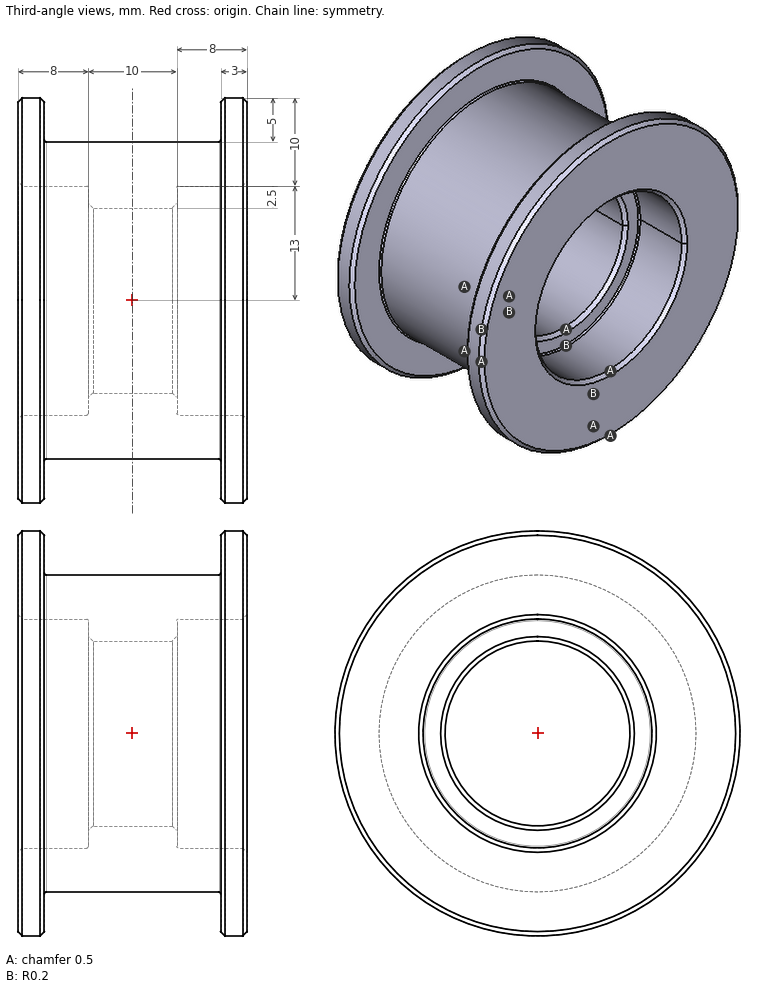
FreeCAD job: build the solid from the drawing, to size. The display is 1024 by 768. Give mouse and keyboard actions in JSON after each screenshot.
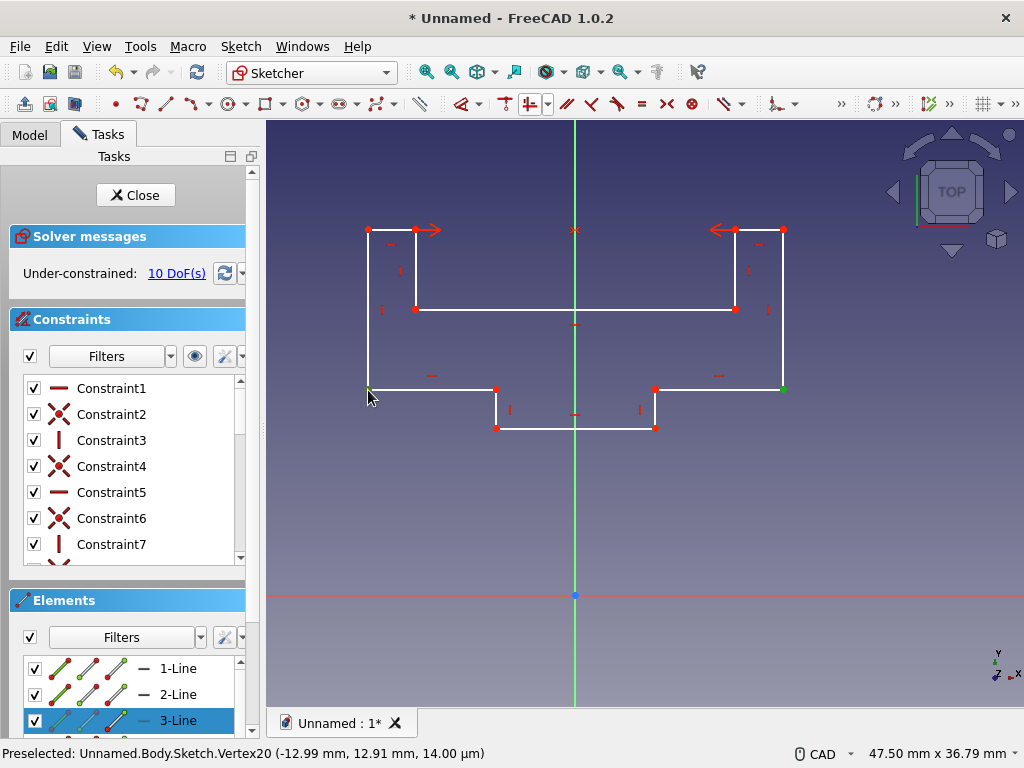
{"action": "left_click", "coordinate": [575, 641]}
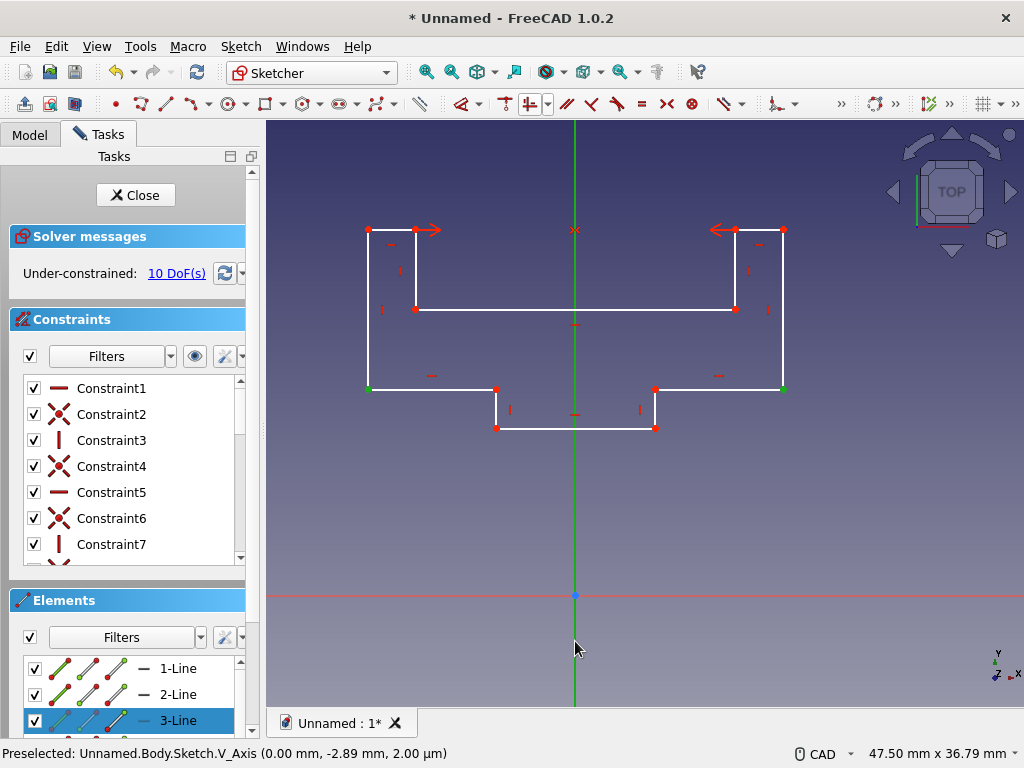
{"action": "left_click", "coordinate": [667, 104]}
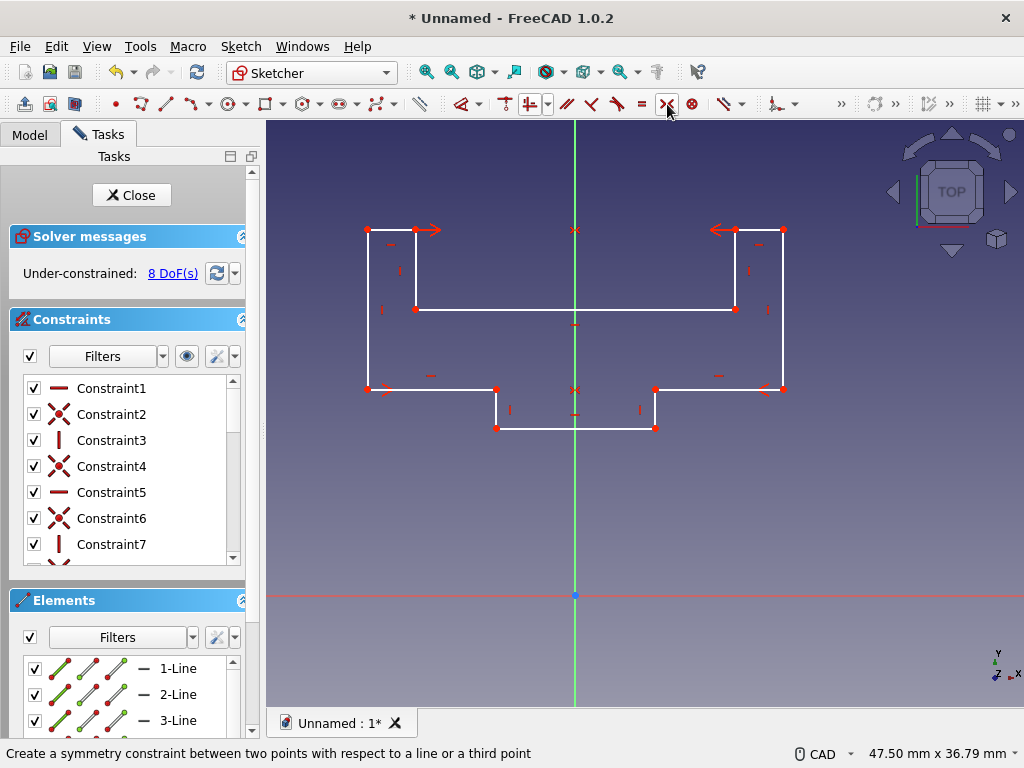
{"action": "left_click", "coordinate": [693, 390]}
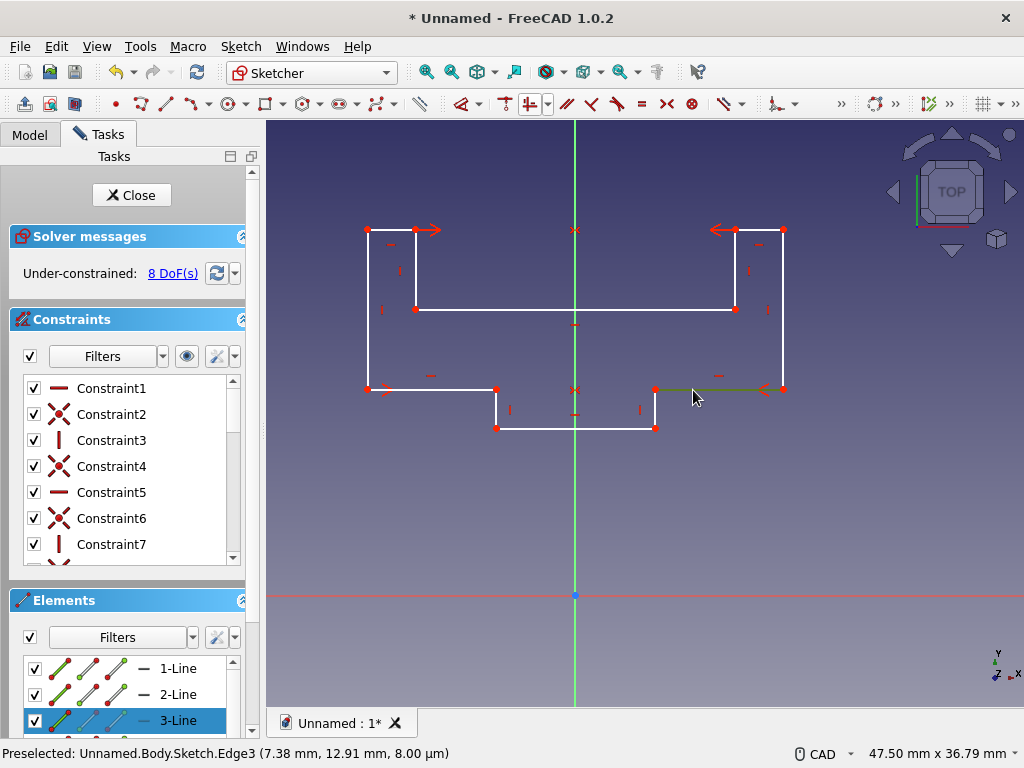
{"action": "left_click", "coordinate": [478, 104]}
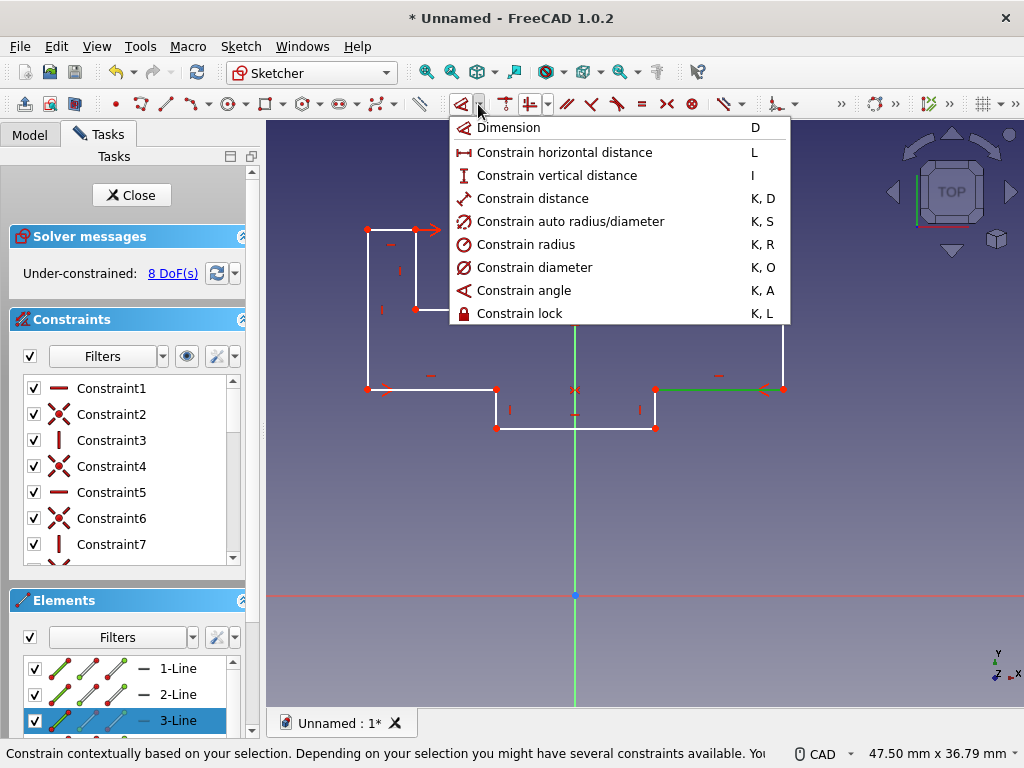
{"action": "left_click", "coordinate": [620, 152]}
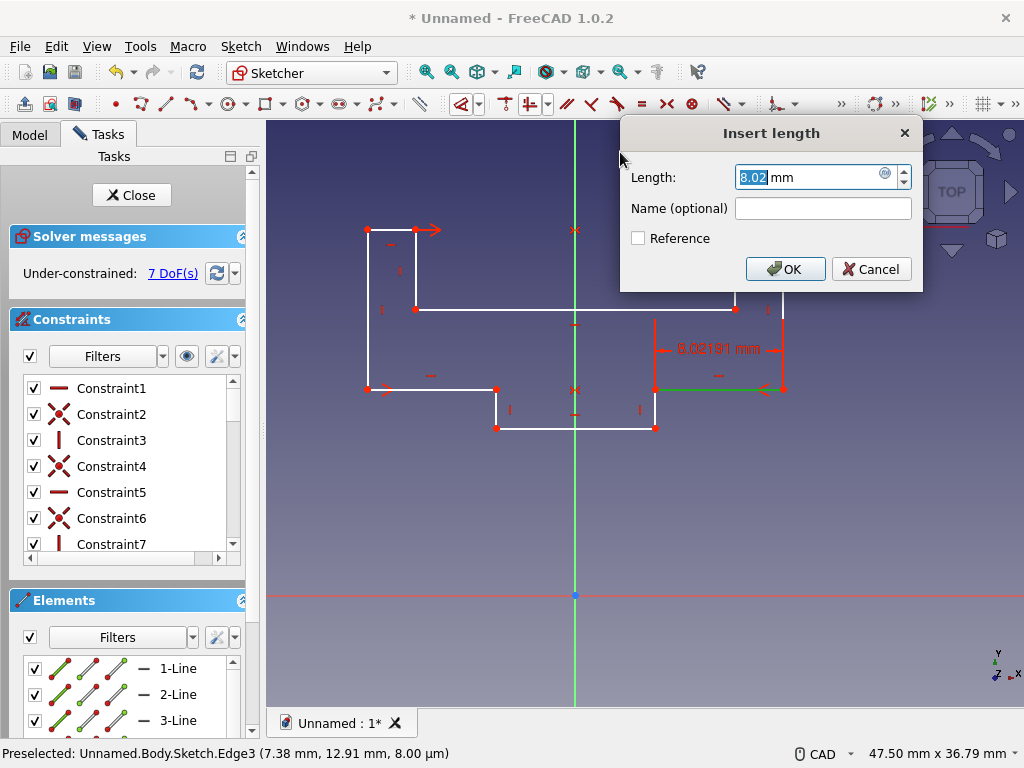
{"action": "type", "text": "8"}
{"action": "key", "text": "Return"}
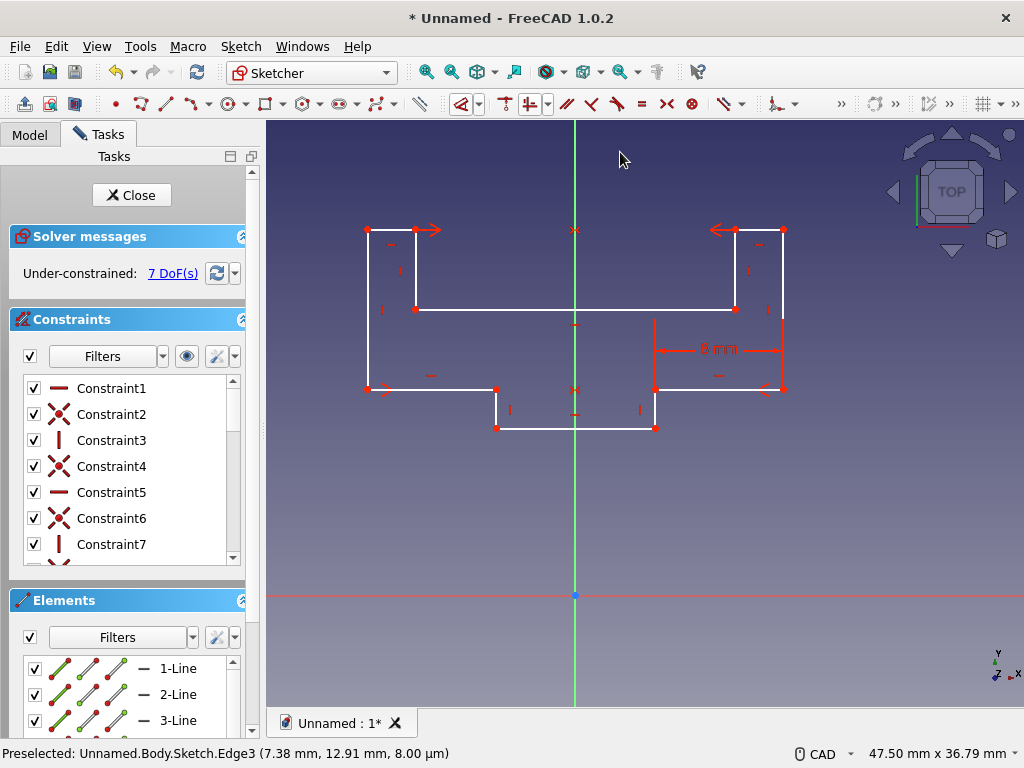
{"action": "left_click", "coordinate": [769, 230]}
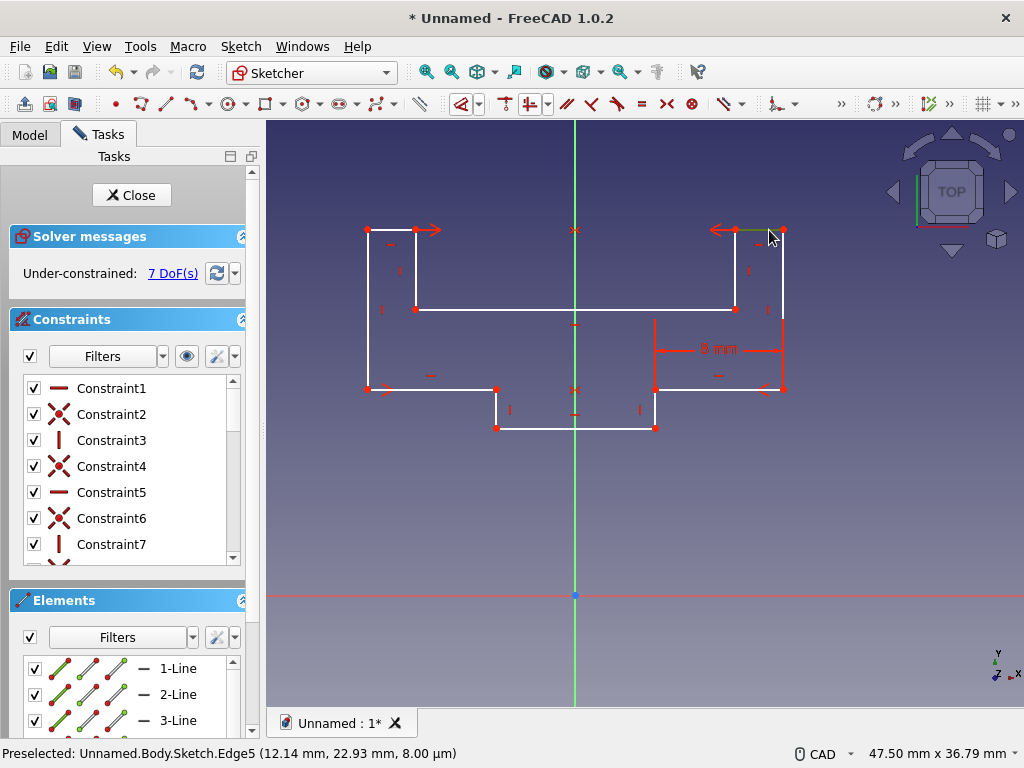
{"action": "key", "text": "l"}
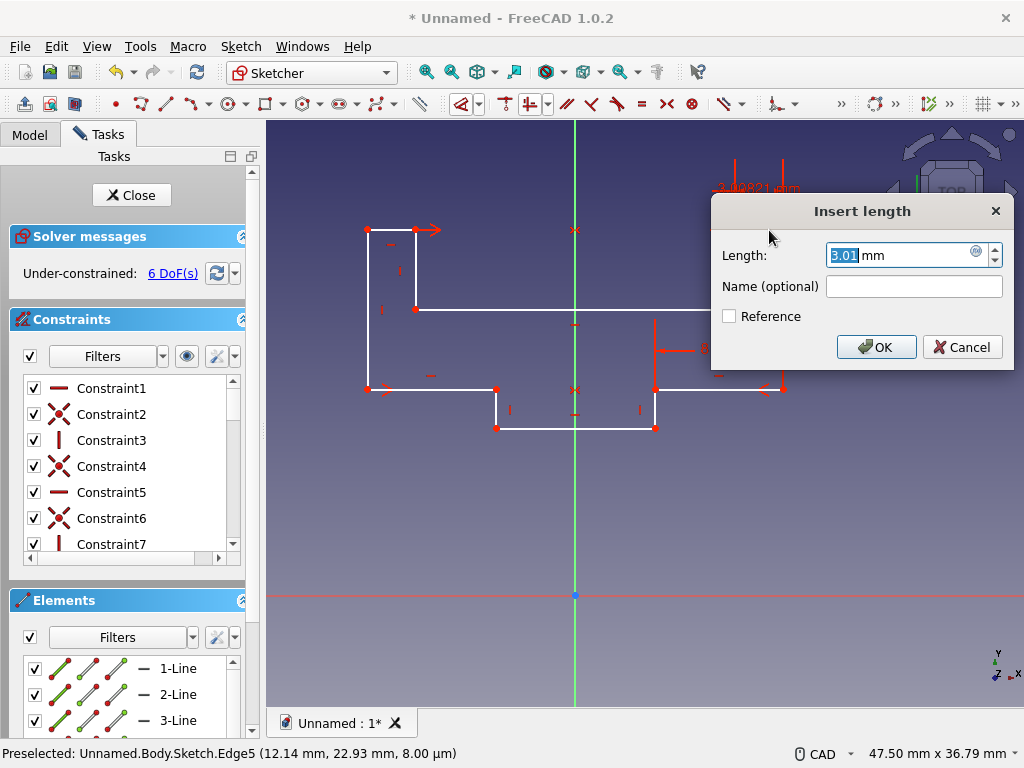
{"action": "type", "text": "3"}
{"action": "key", "text": "Return"}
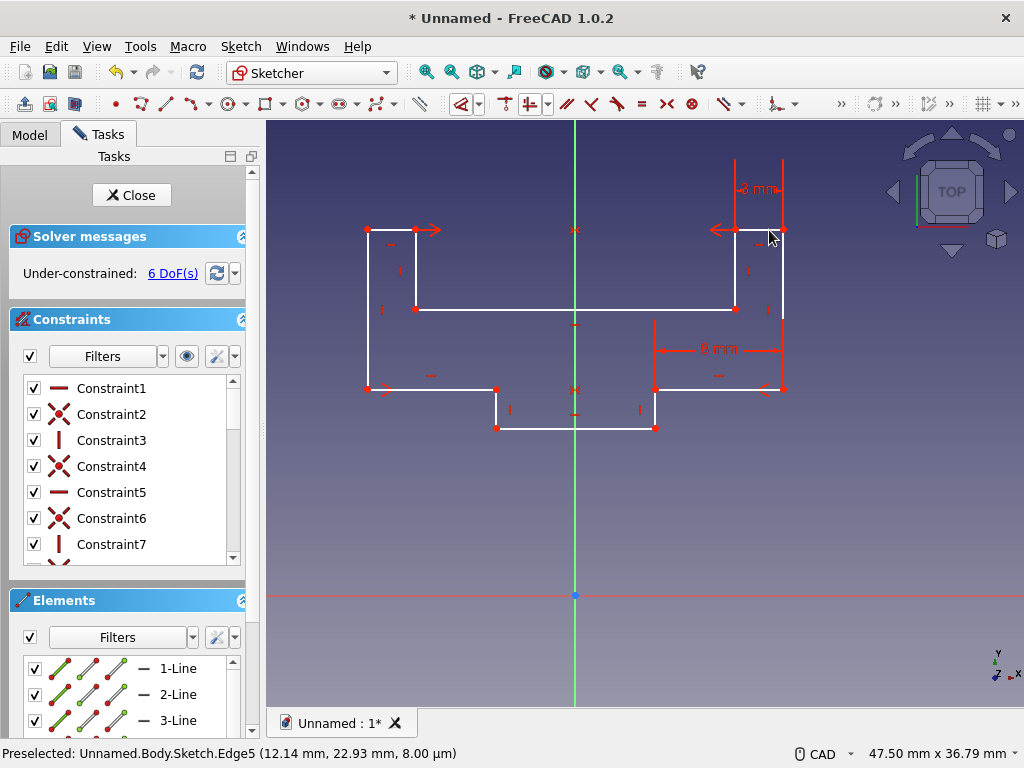
{"action": "left_click", "coordinate": [735, 254]}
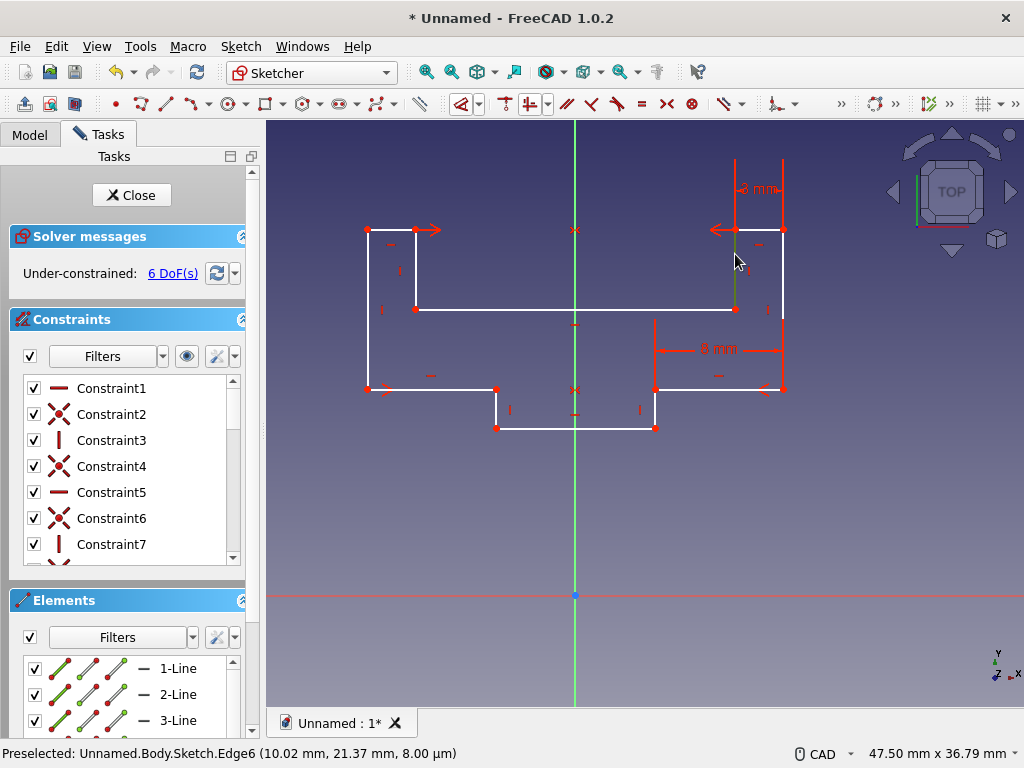
{"action": "left_click", "coordinate": [478, 104]}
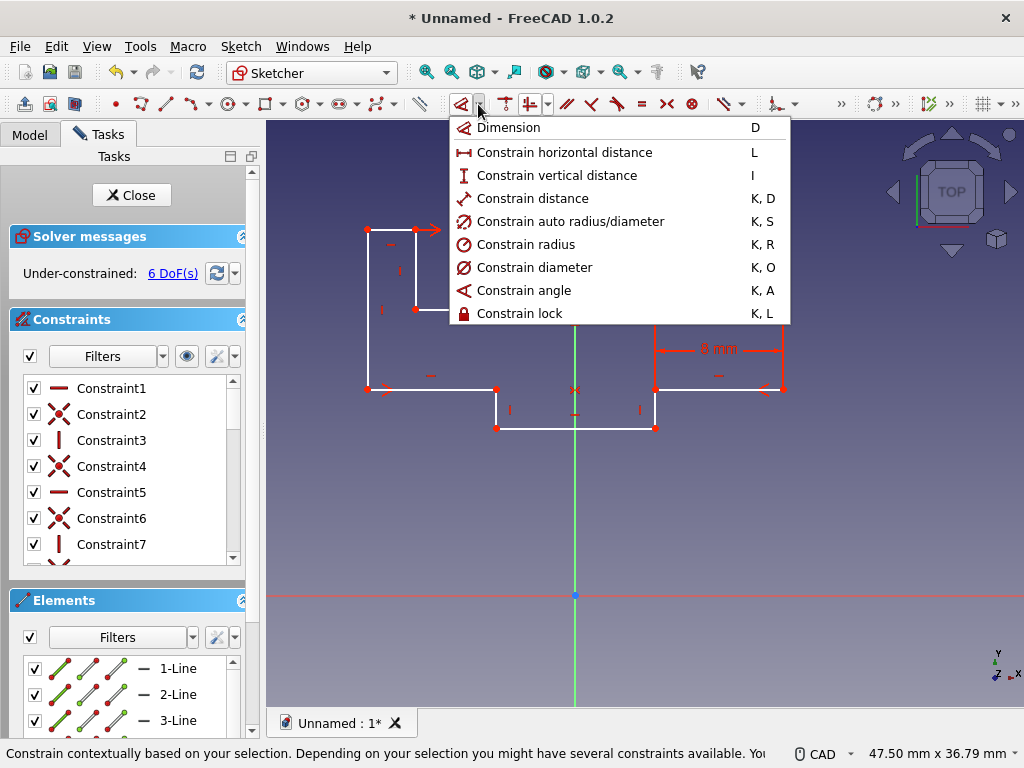
{"action": "left_click", "coordinate": [620, 176]}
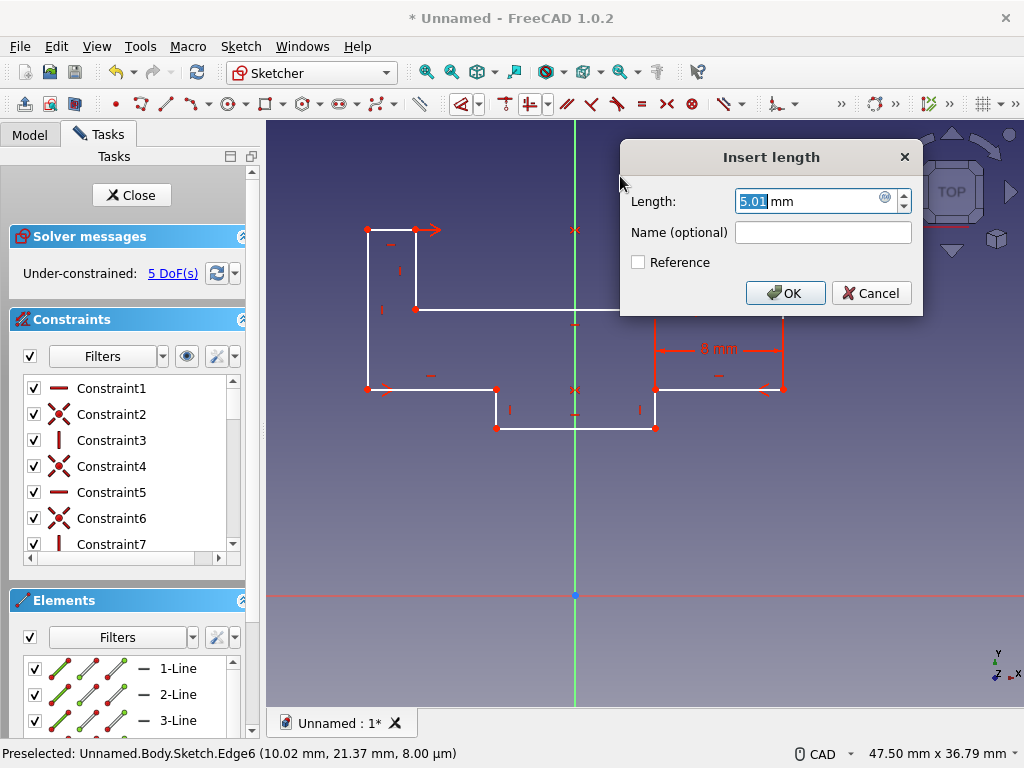
{"action": "type", "text": "5"}
{"action": "key", "text": "Return"}